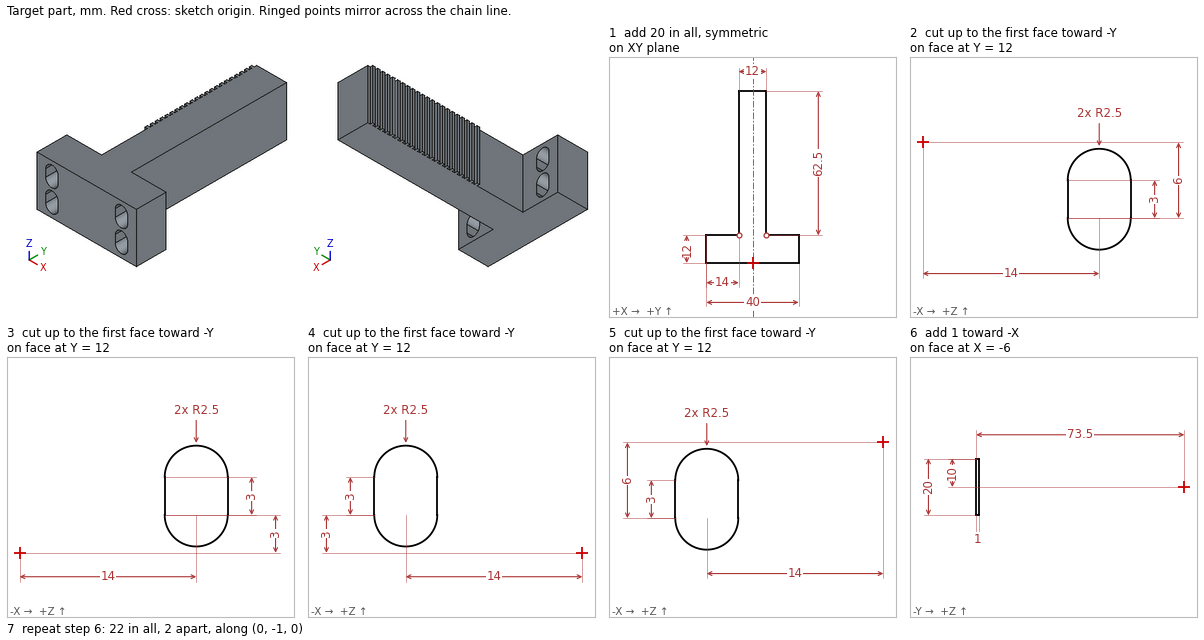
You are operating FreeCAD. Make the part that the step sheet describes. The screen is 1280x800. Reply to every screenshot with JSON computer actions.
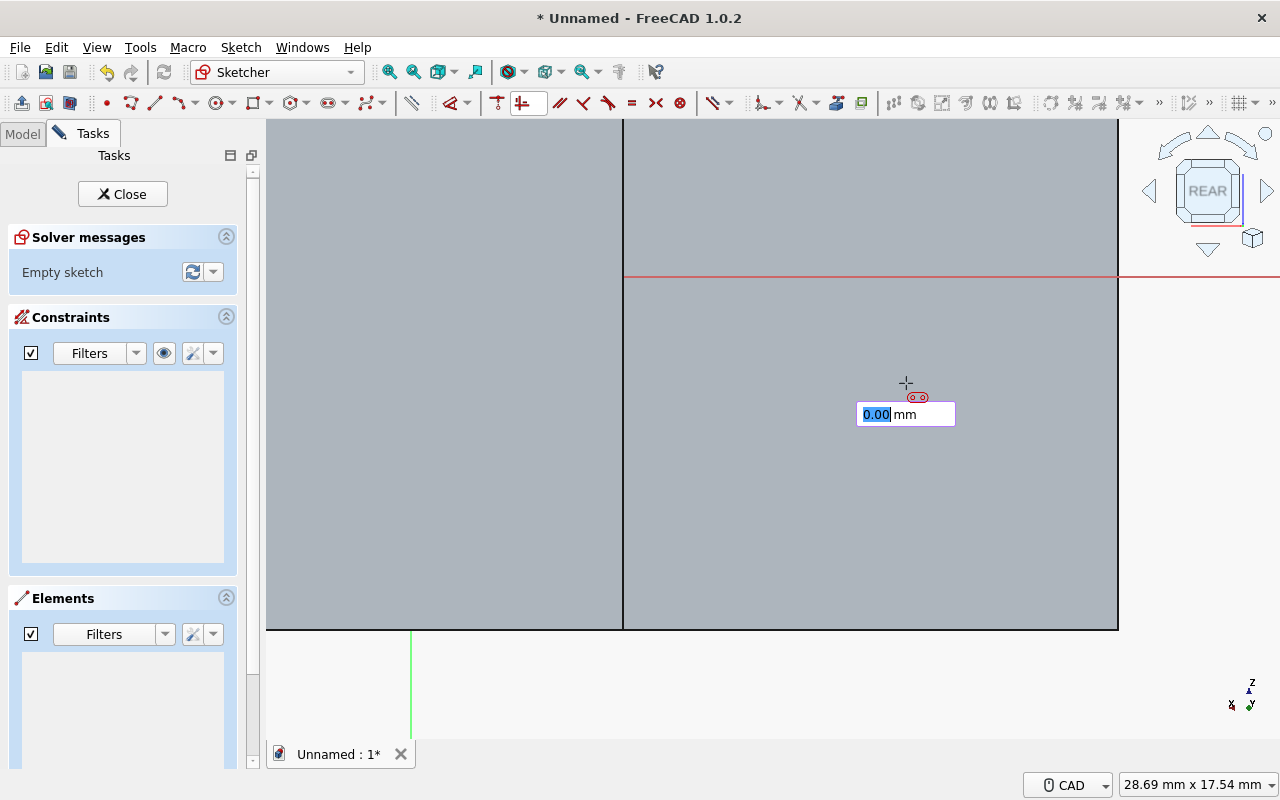
{"action": "left_click", "coordinate": [994, 436]}
{"action": "key", "text": "Escape"}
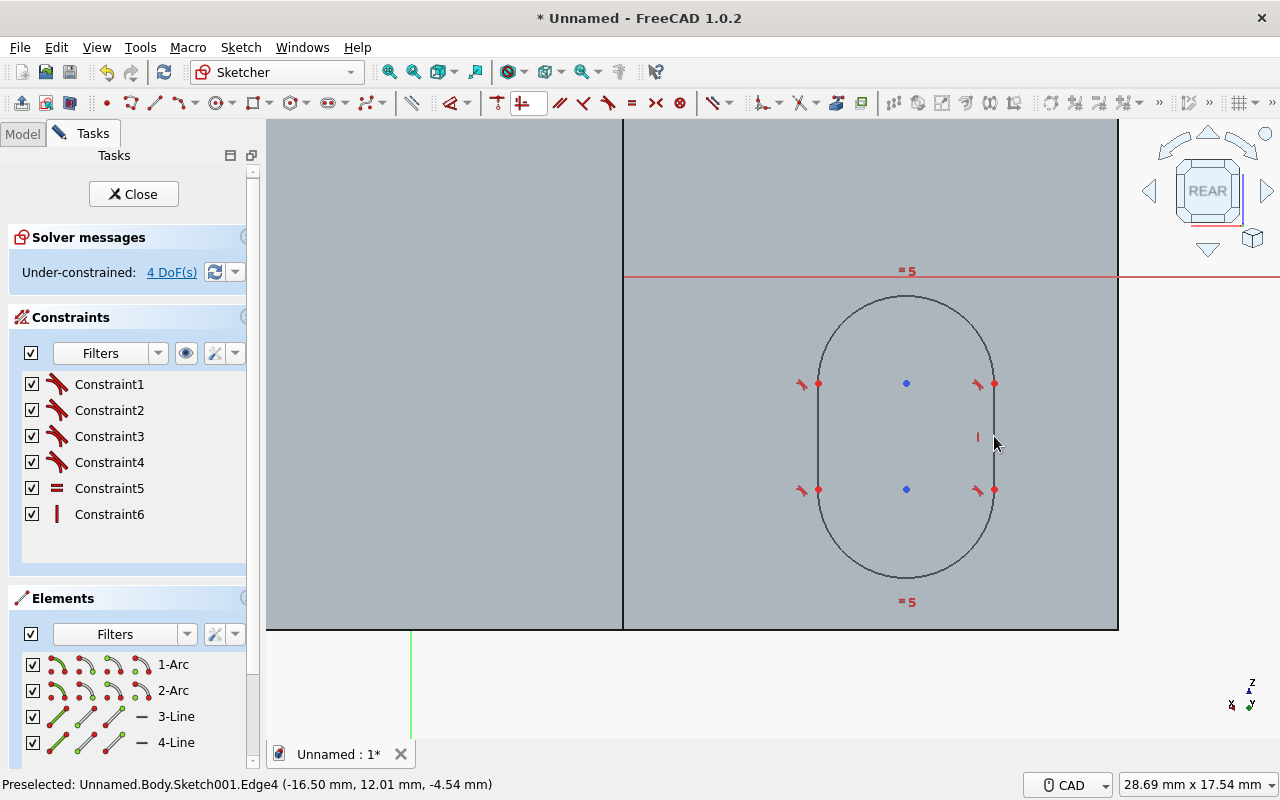
{"action": "left_click", "coordinate": [450, 104]}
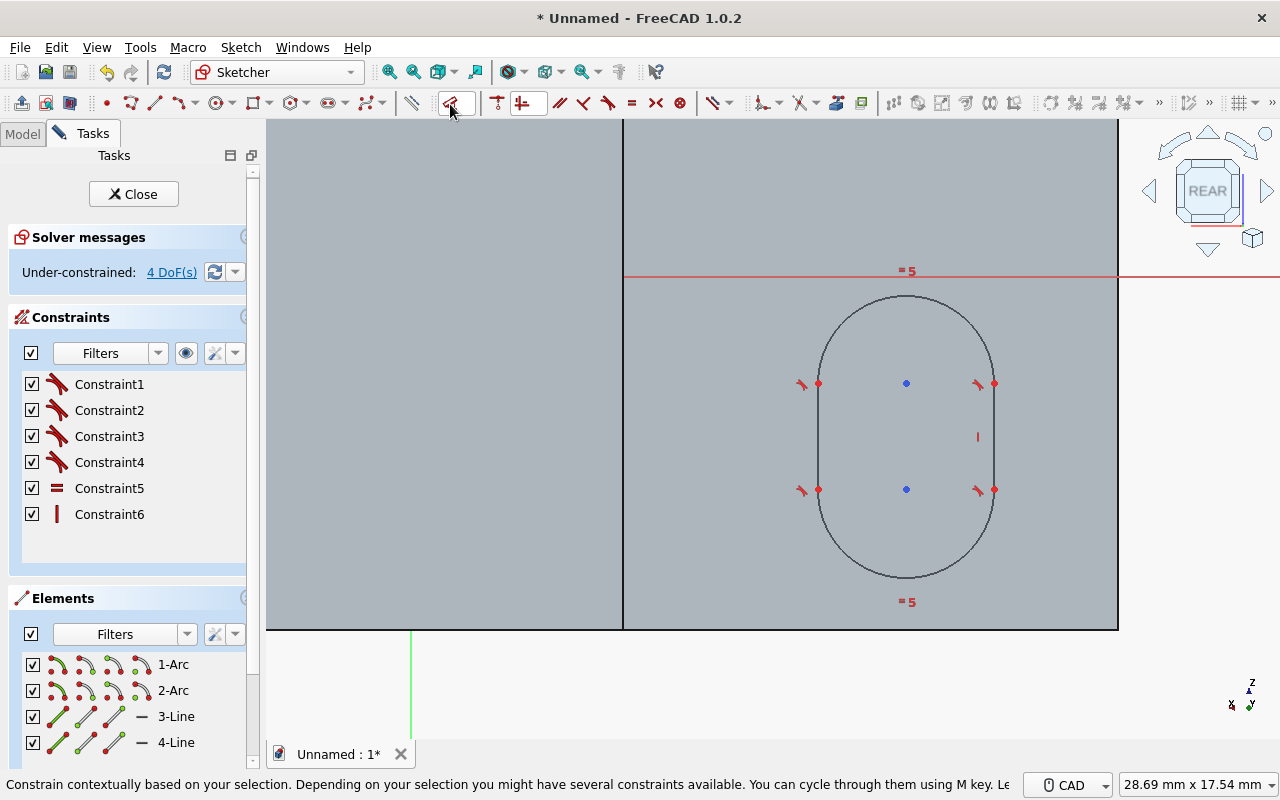
{"action": "left_click", "coordinate": [854, 561]}
{"action": "left_click", "coordinate": [835, 587]}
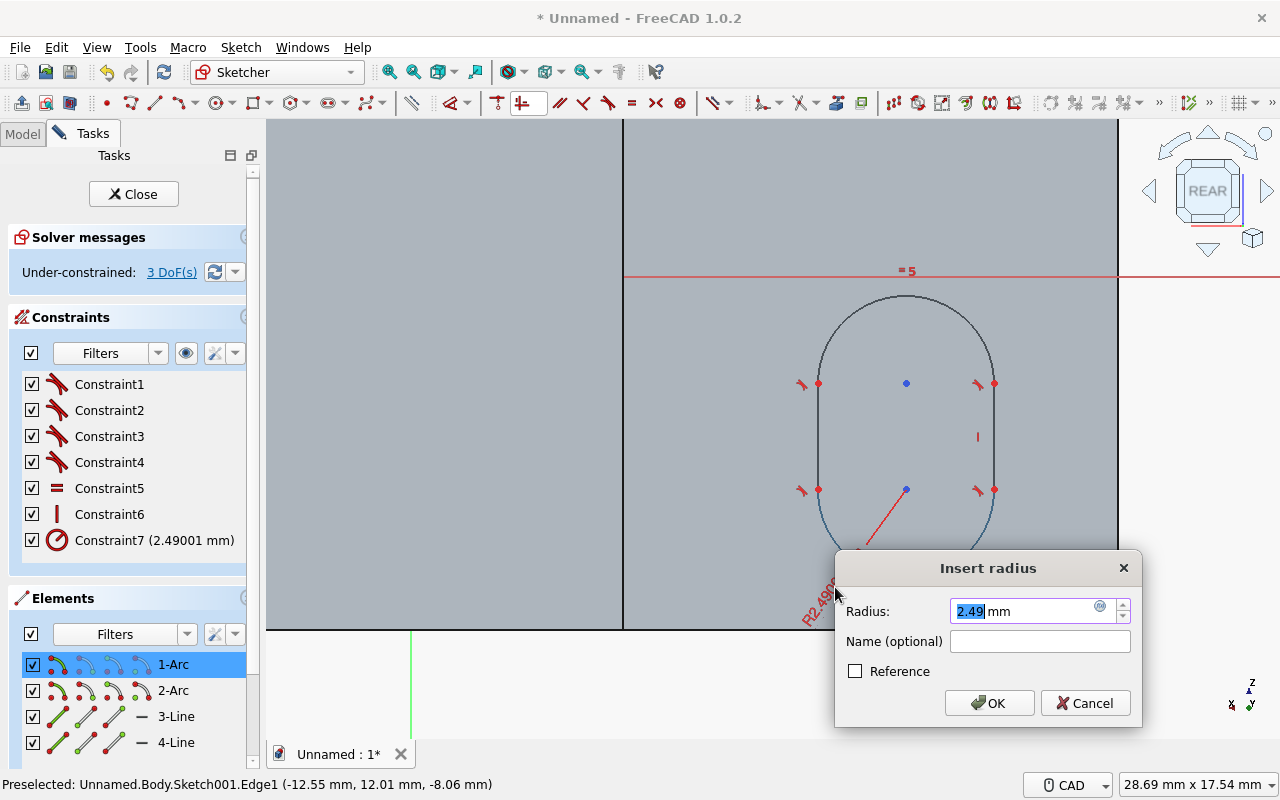
{"action": "type", "text": "2.5"}
{"action": "key", "text": "Return"}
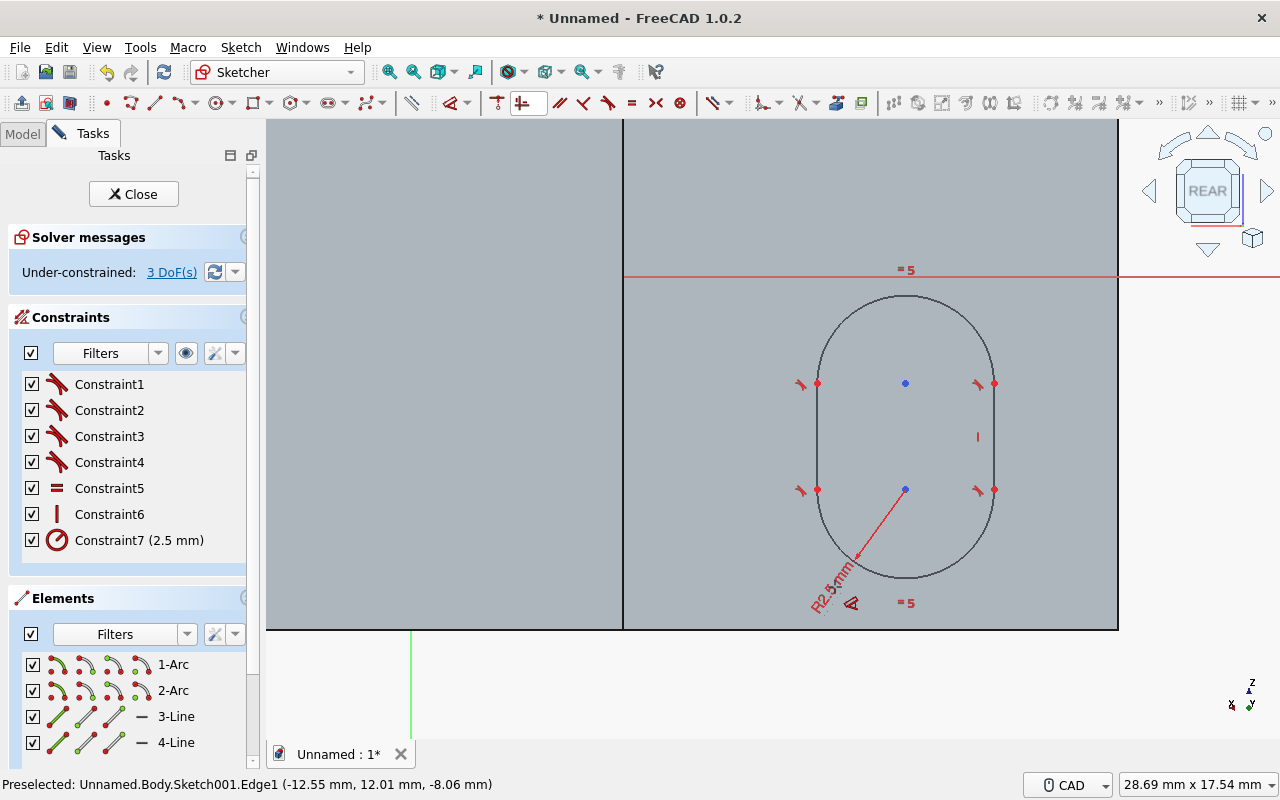
{"action": "left_click", "coordinate": [817, 458]}
{"action": "left_click", "coordinate": [851, 437]}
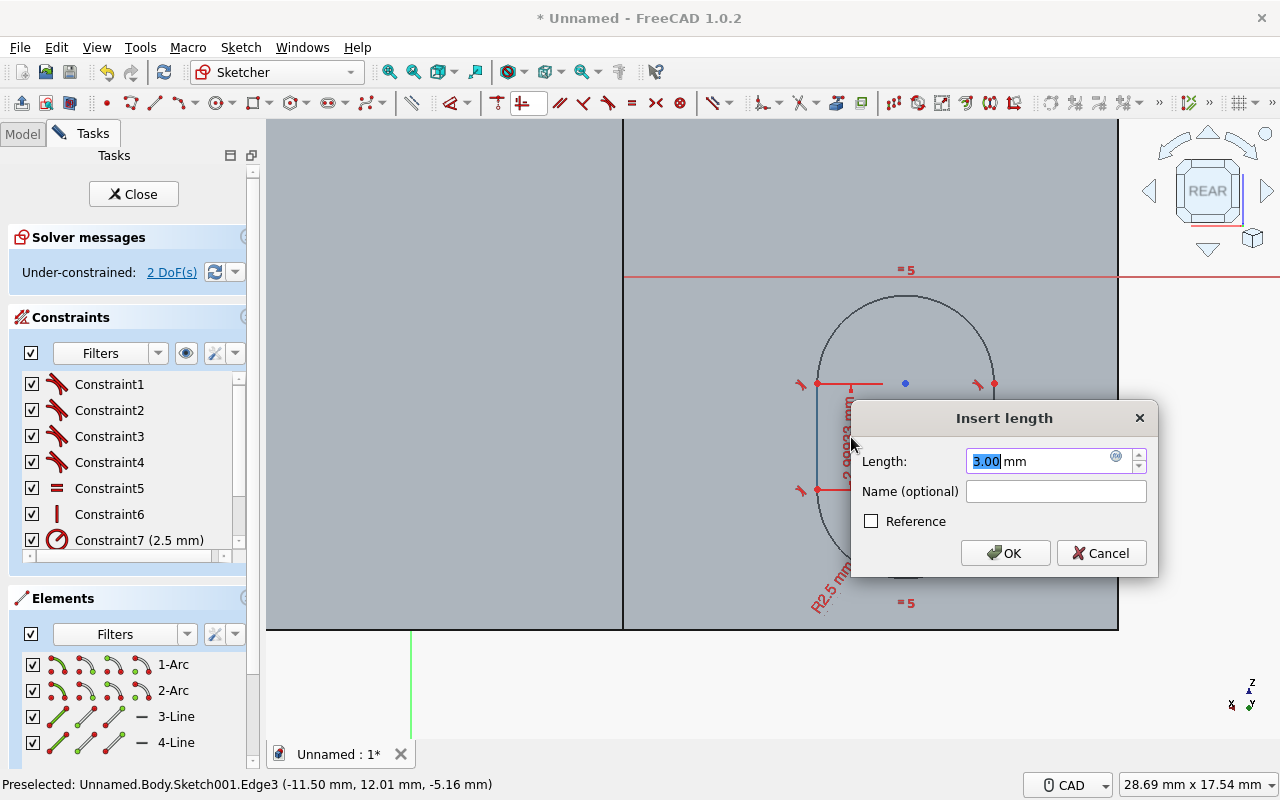
{"action": "type", "text": "3"}
{"action": "key", "text": "Return"}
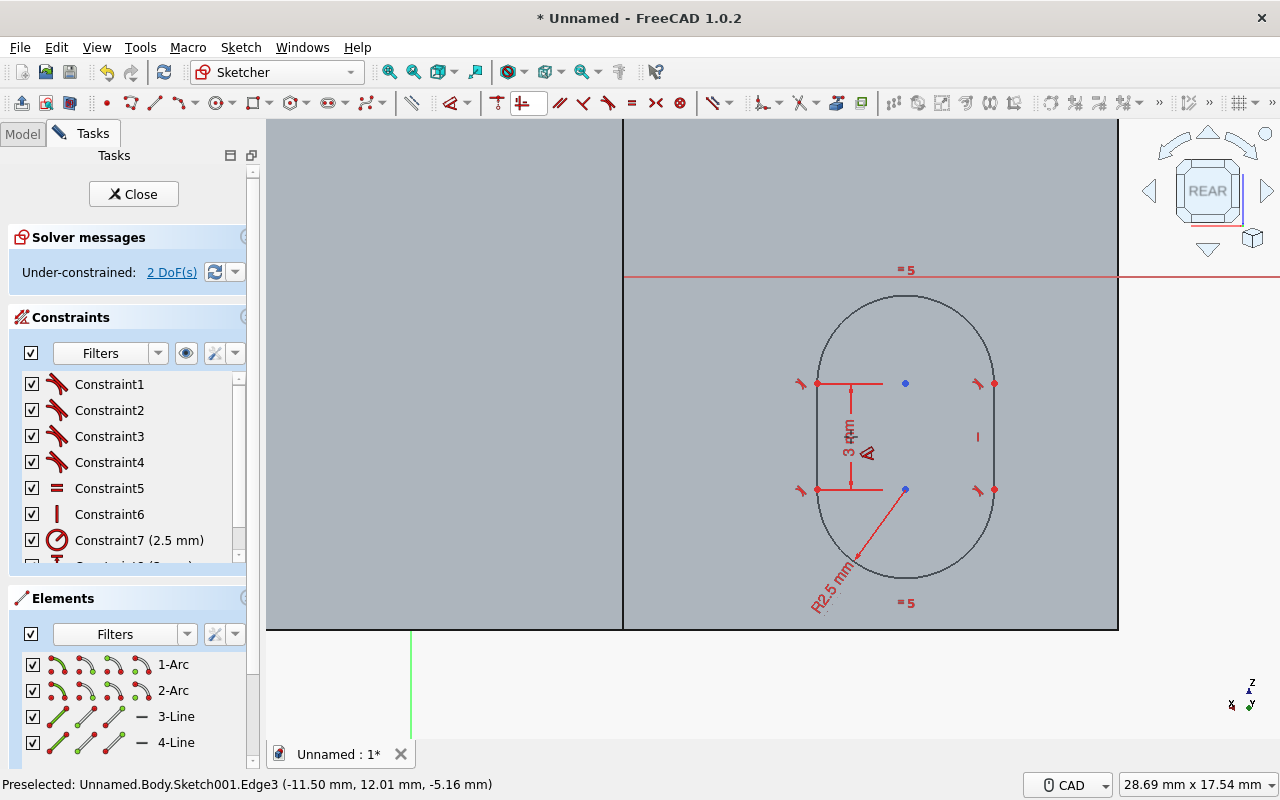
{"action": "left_click", "coordinate": [817, 490]}
{"action": "left_click", "coordinate": [377, 383]}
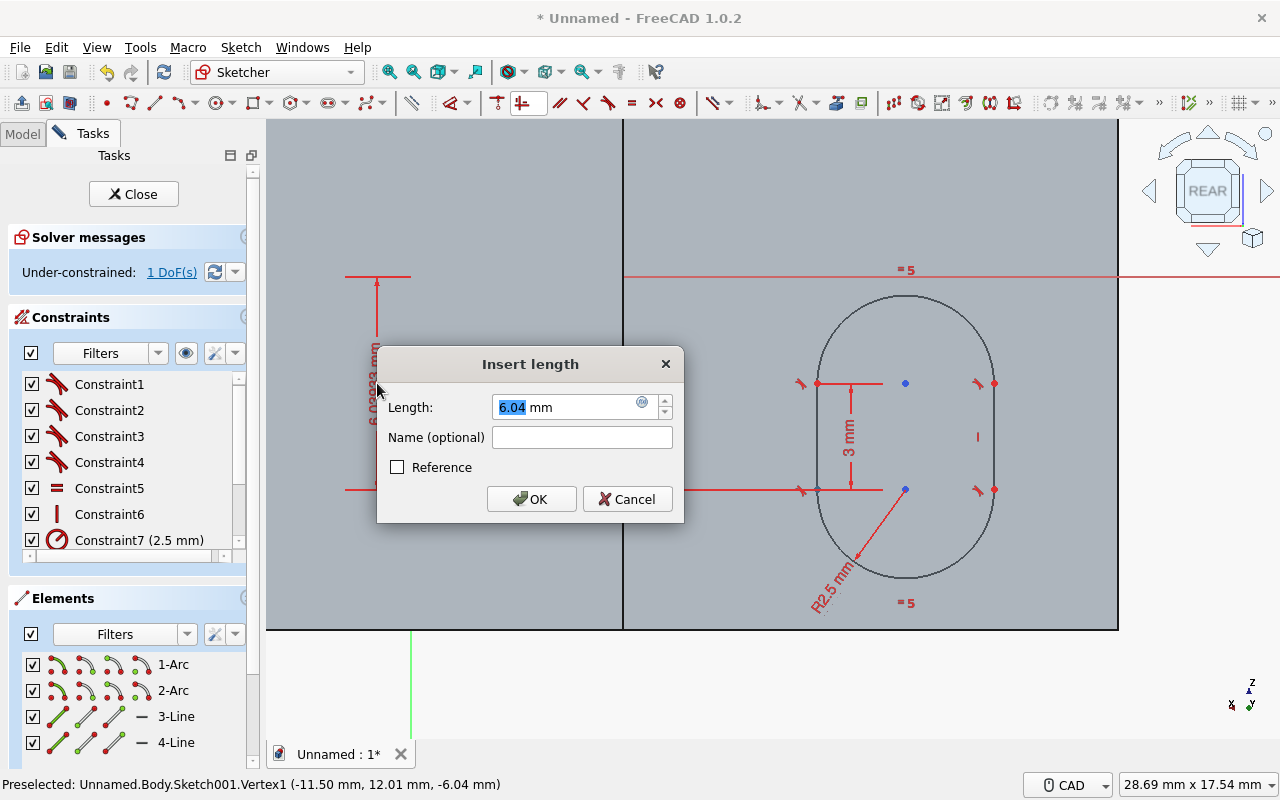
{"action": "type", "text": "6"}
{"action": "key", "text": "Return"}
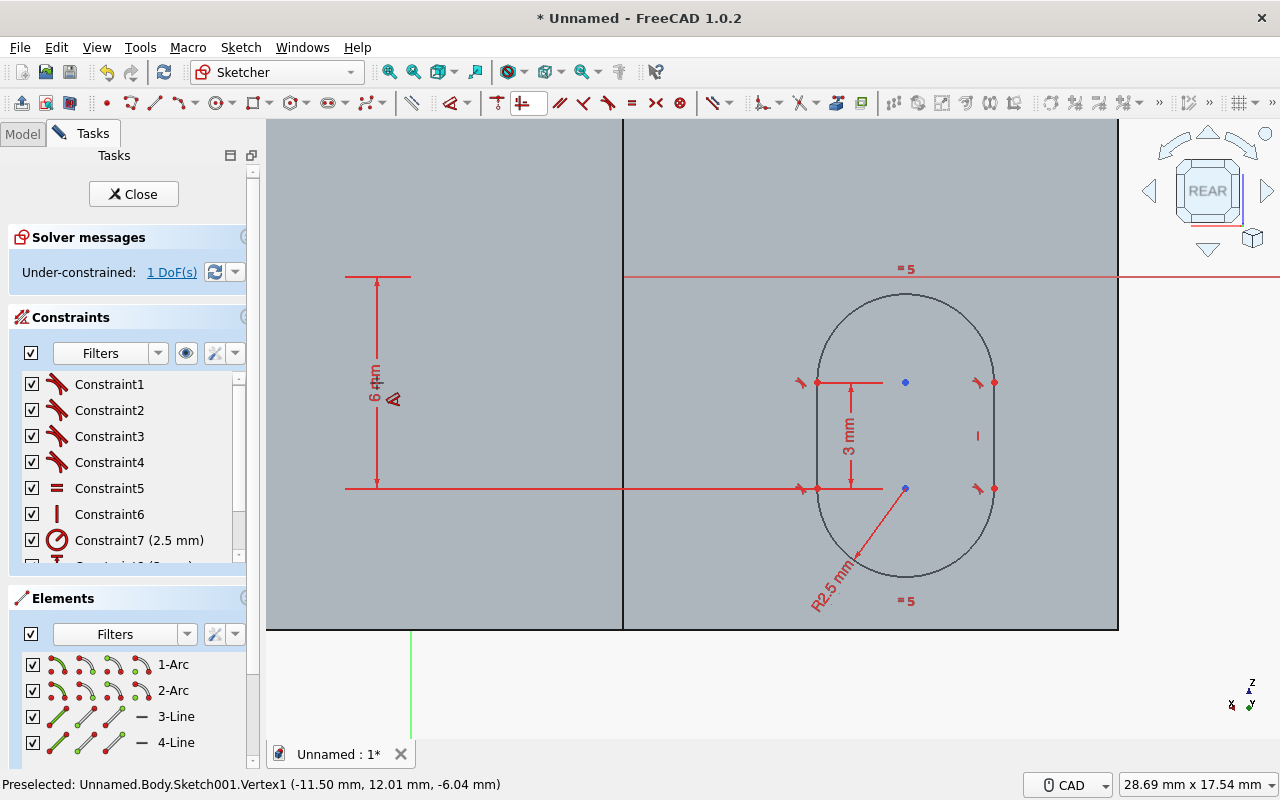
{"action": "left_click", "coordinate": [906, 489]}
{"action": "left_click", "coordinate": [658, 243]}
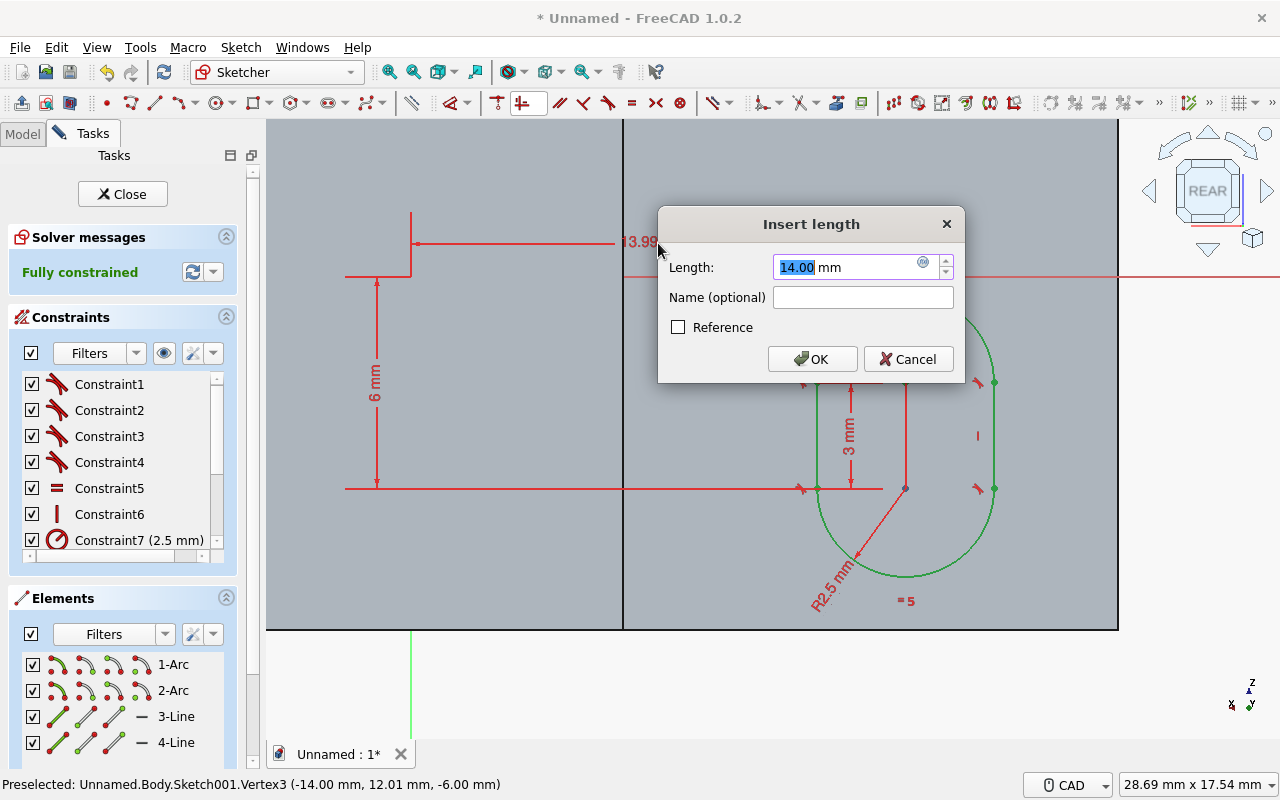
{"action": "type", "text": "14"}
{"action": "key", "text": "Return"}
{"action": "key", "text": "Escape"}